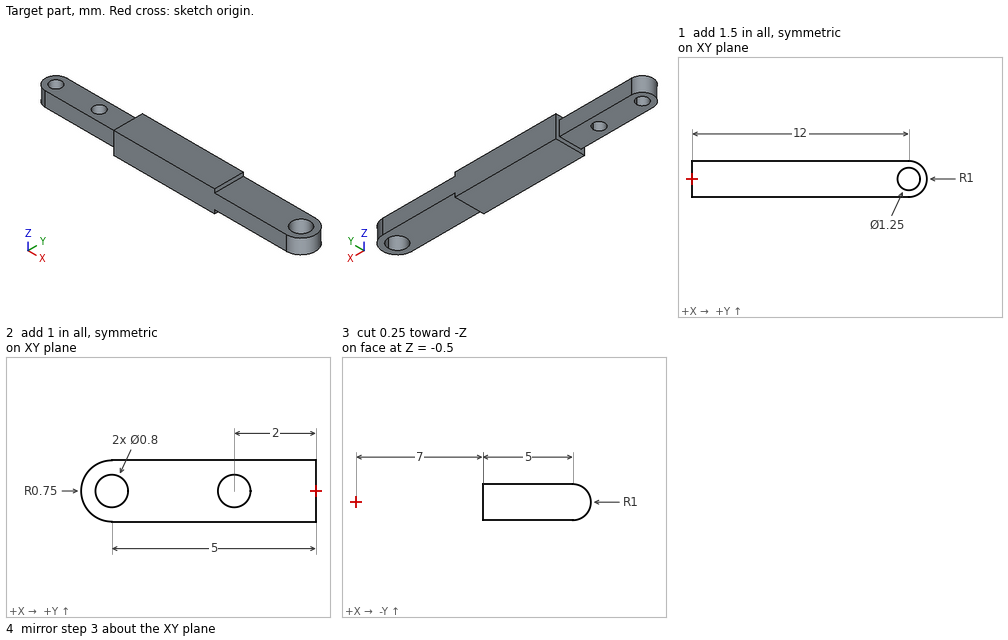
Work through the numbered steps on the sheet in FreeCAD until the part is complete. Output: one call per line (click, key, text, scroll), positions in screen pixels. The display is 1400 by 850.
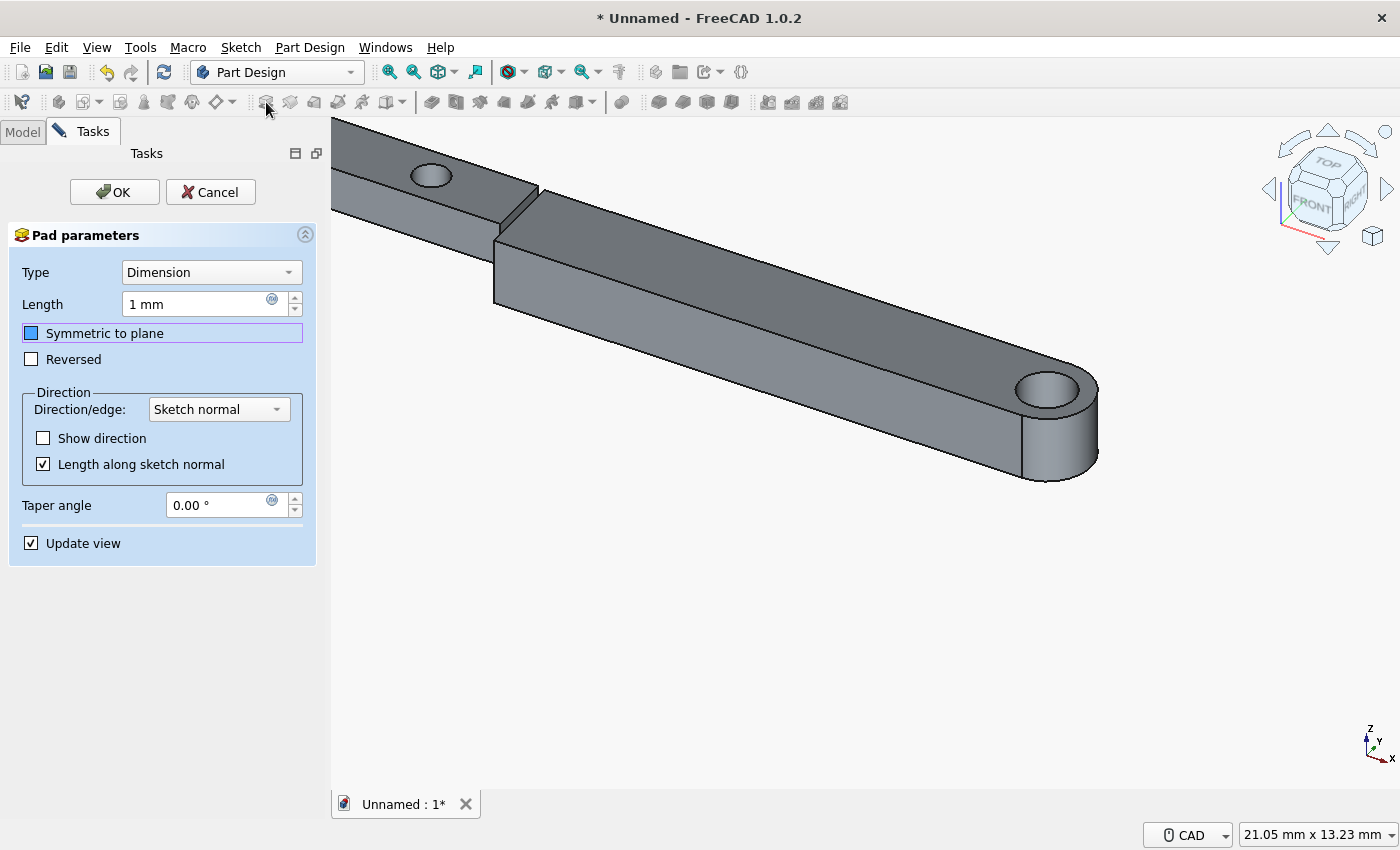
click(30, 333)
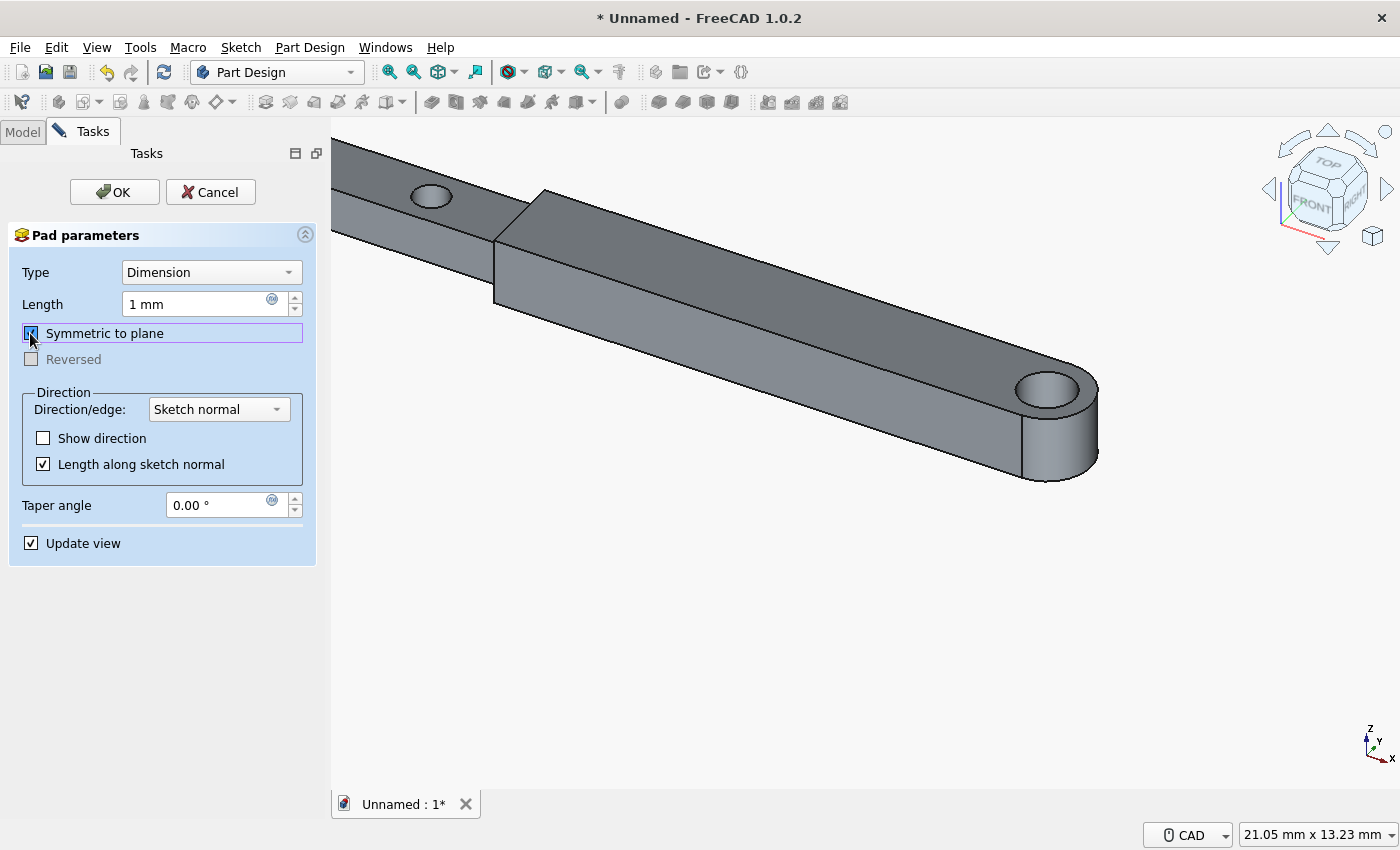
click(115, 192)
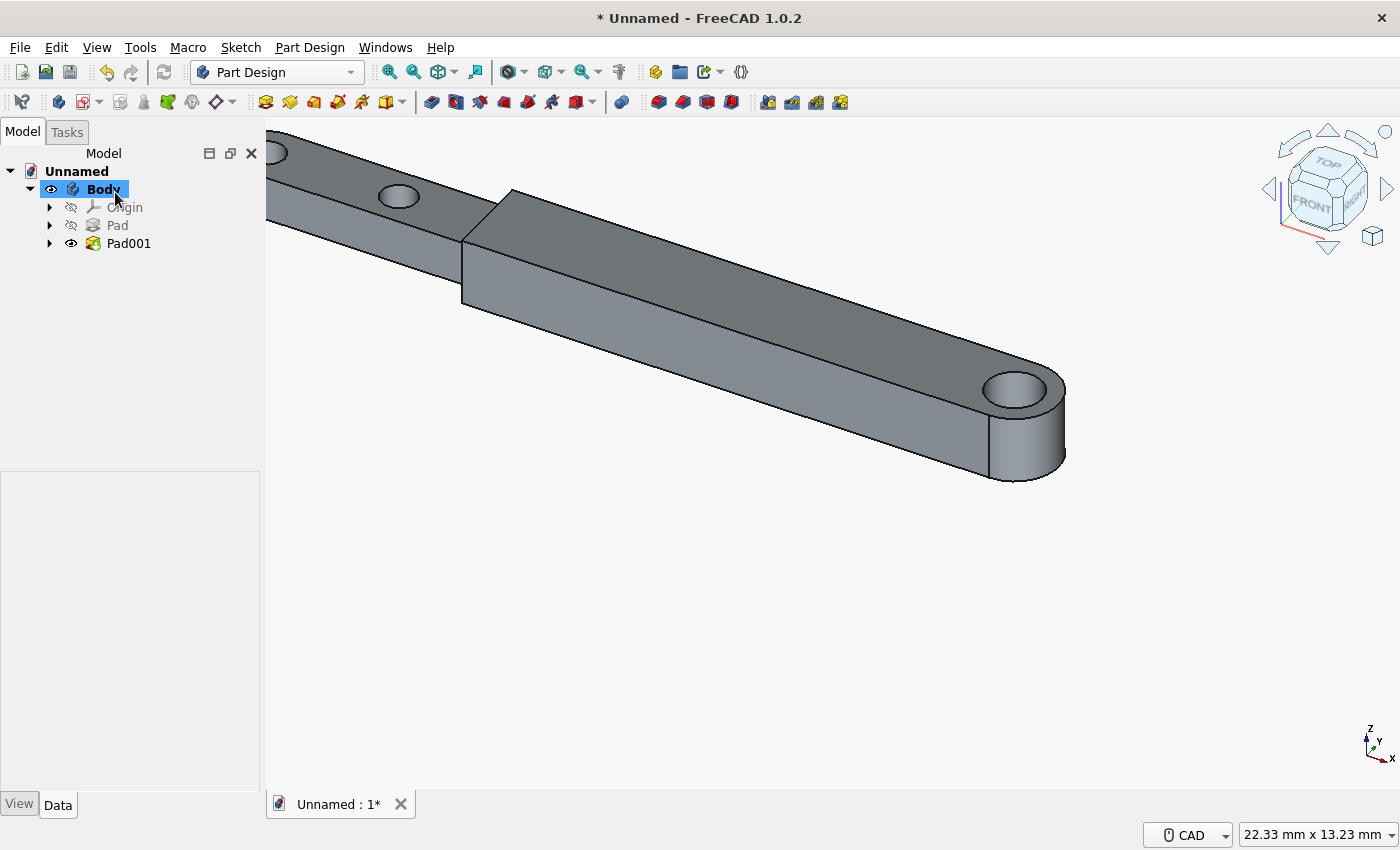
click(390, 72)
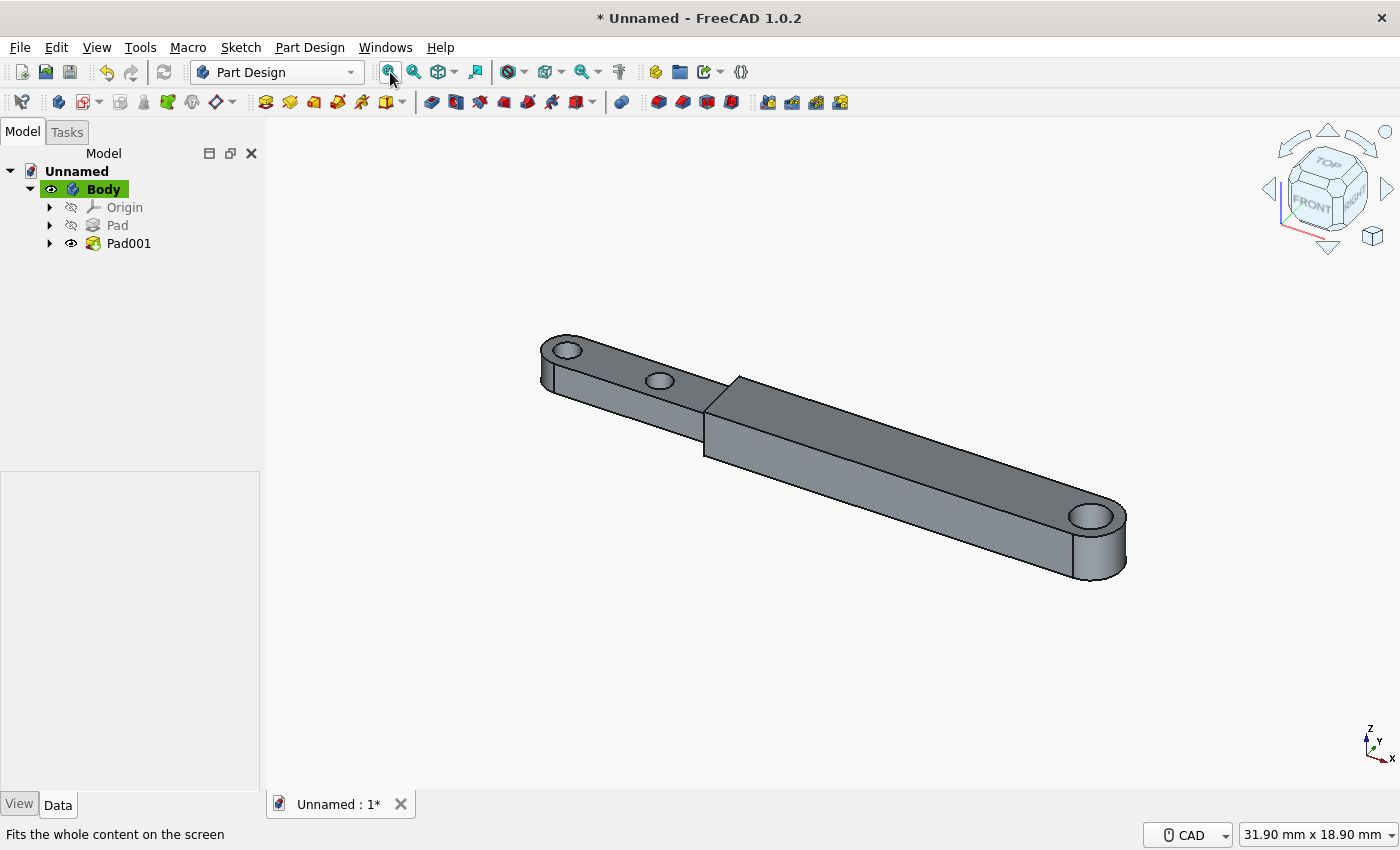
key(5)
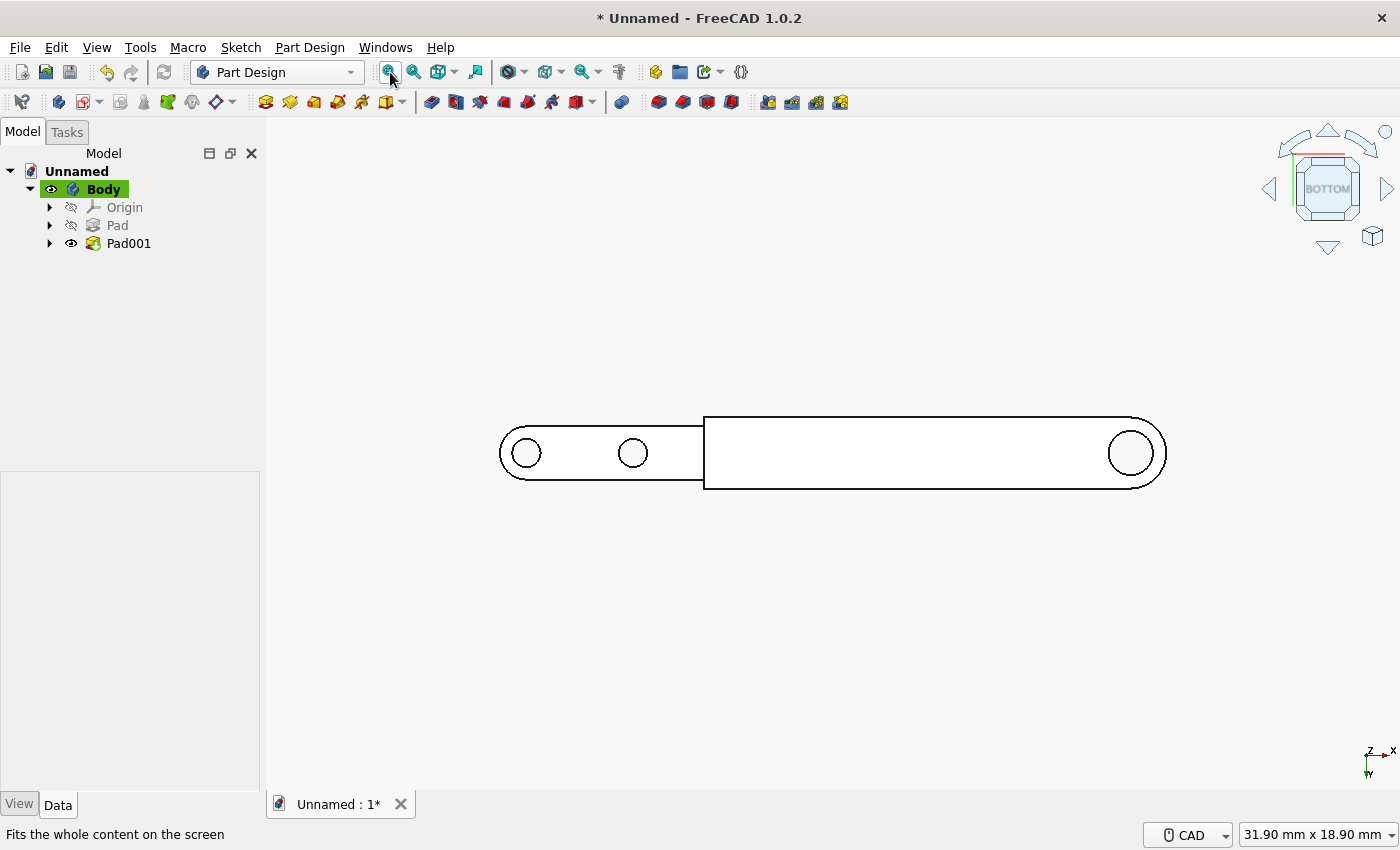
click(573, 452)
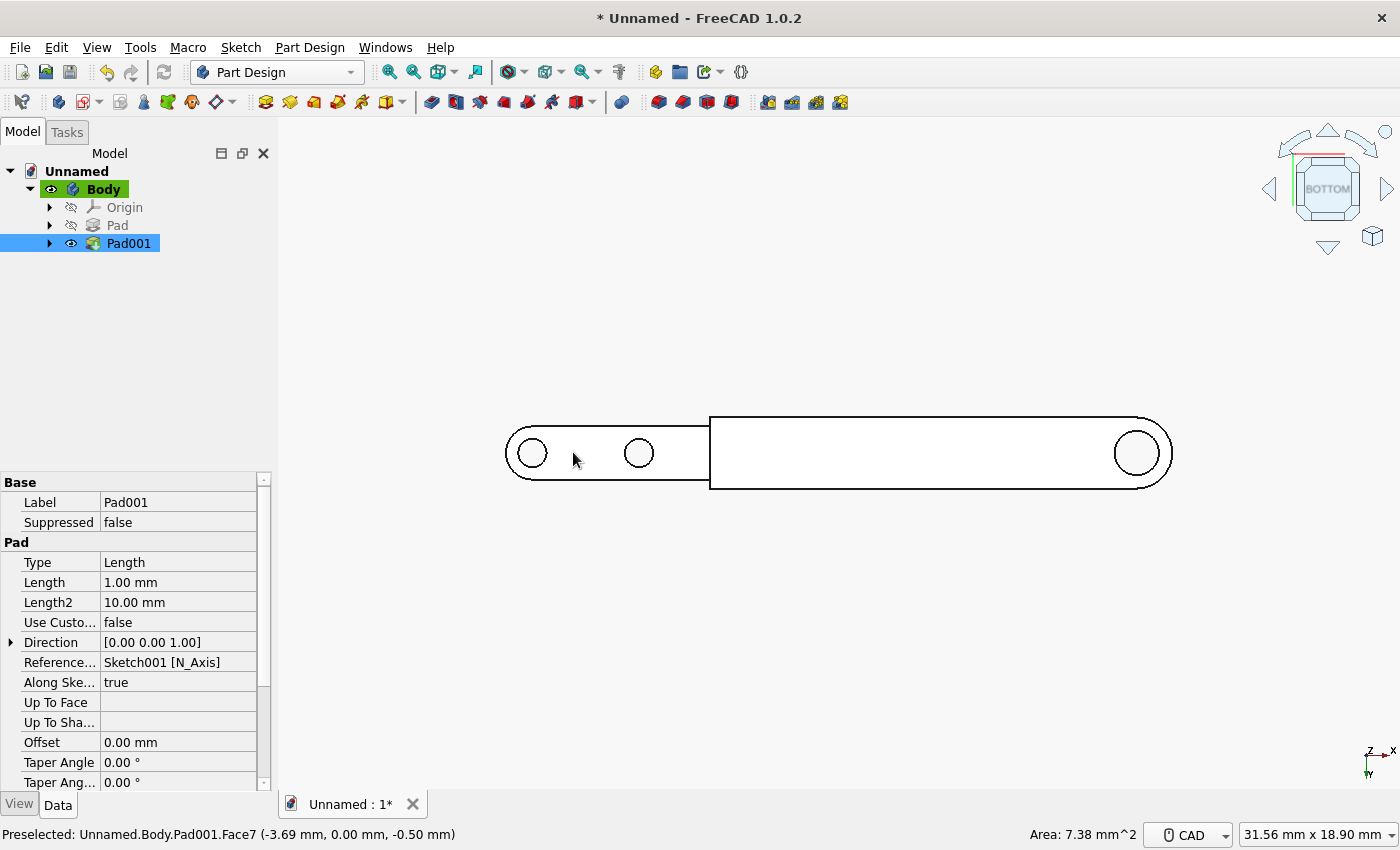
click(84, 102)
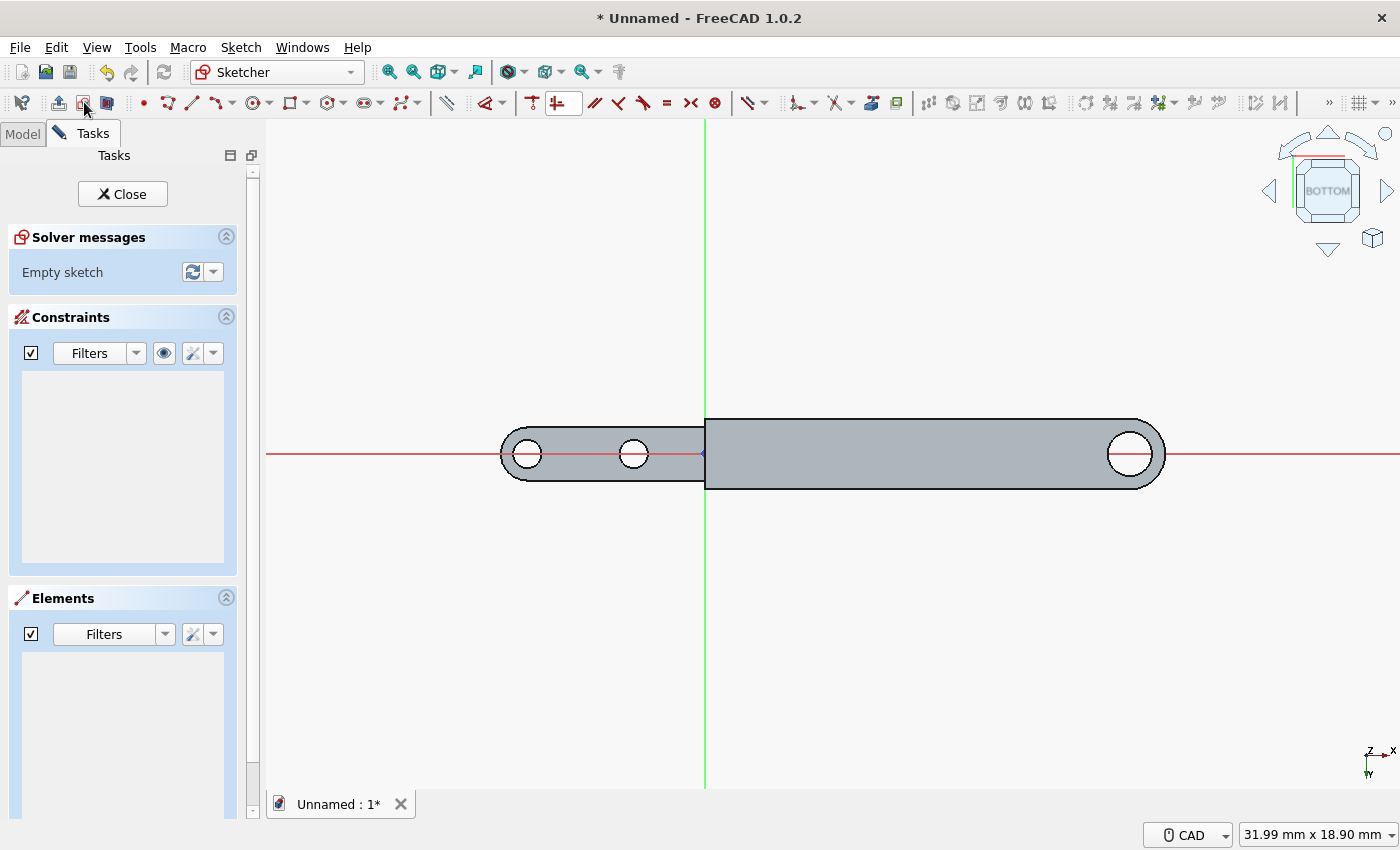
scroll(1235, 454, up, 2)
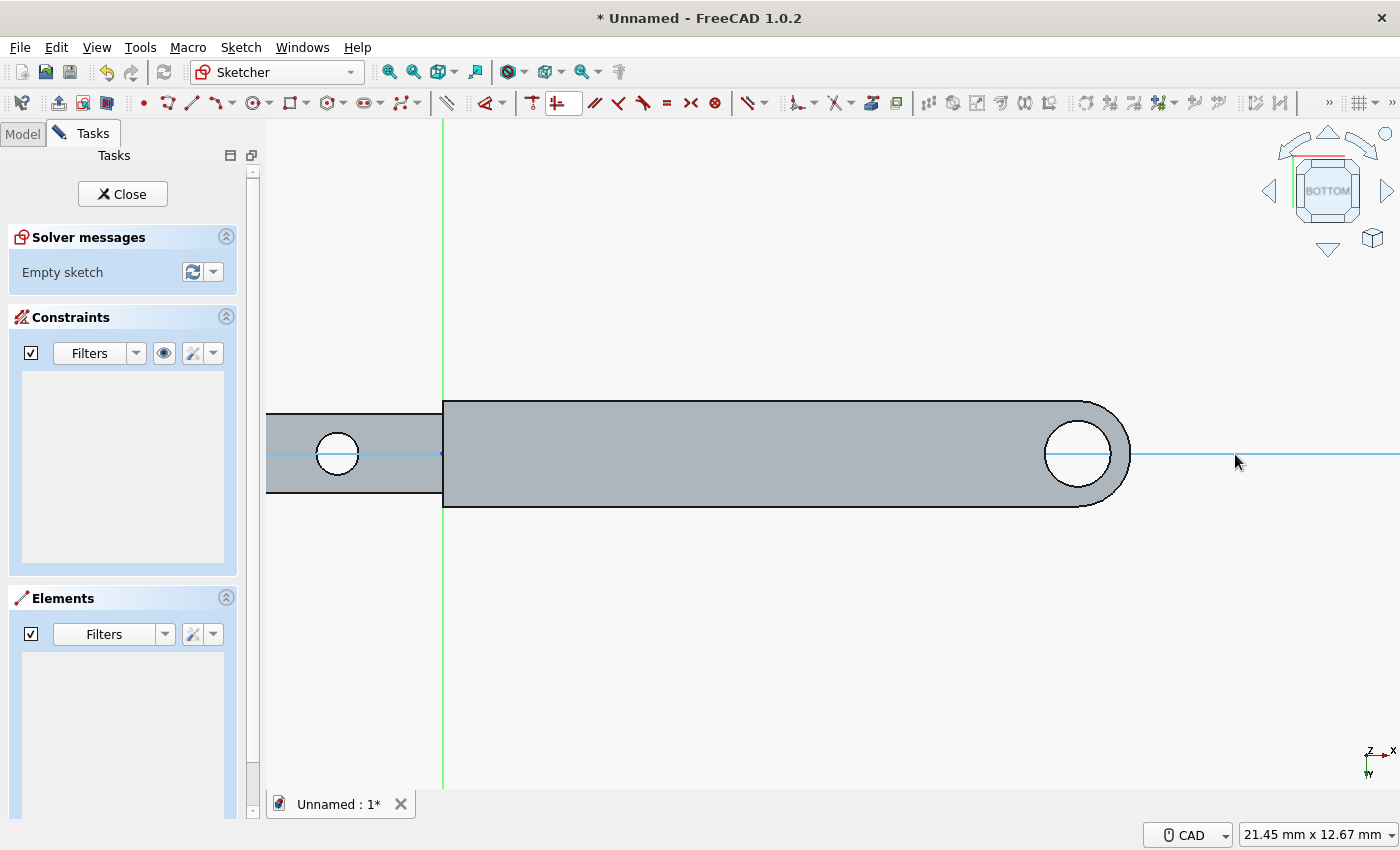
click(168, 104)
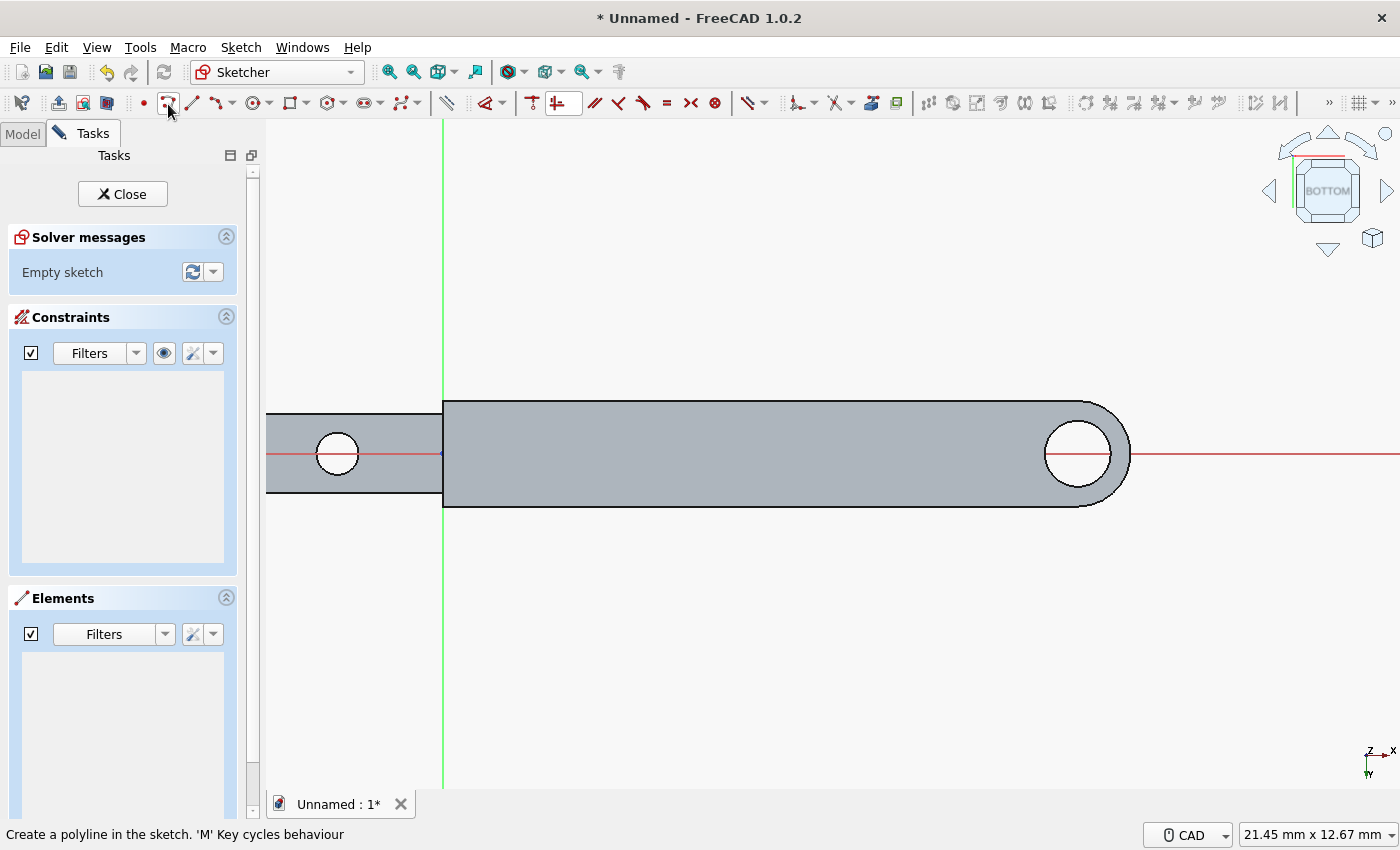
click(1078, 401)
click(813, 401)
click(813, 507)
click(1078, 507)
right_click(1078, 507)